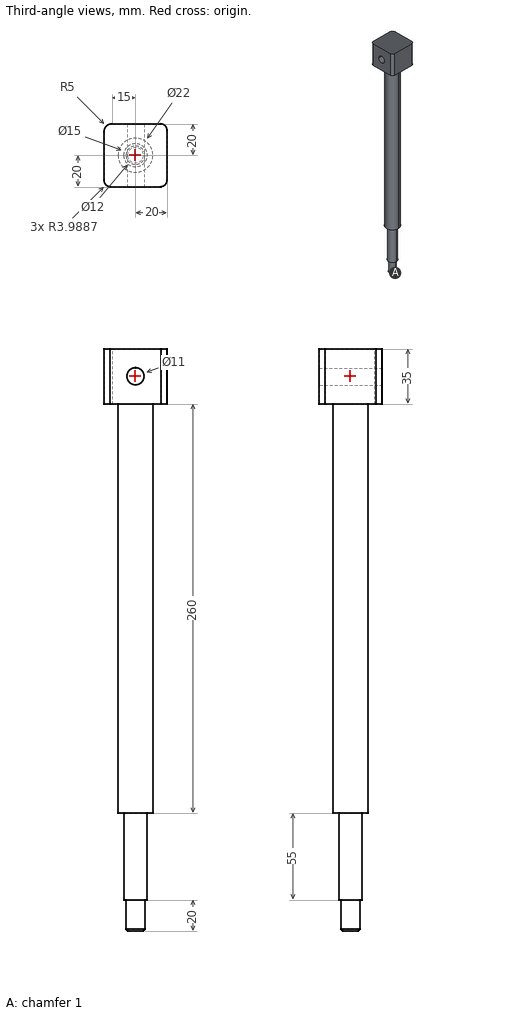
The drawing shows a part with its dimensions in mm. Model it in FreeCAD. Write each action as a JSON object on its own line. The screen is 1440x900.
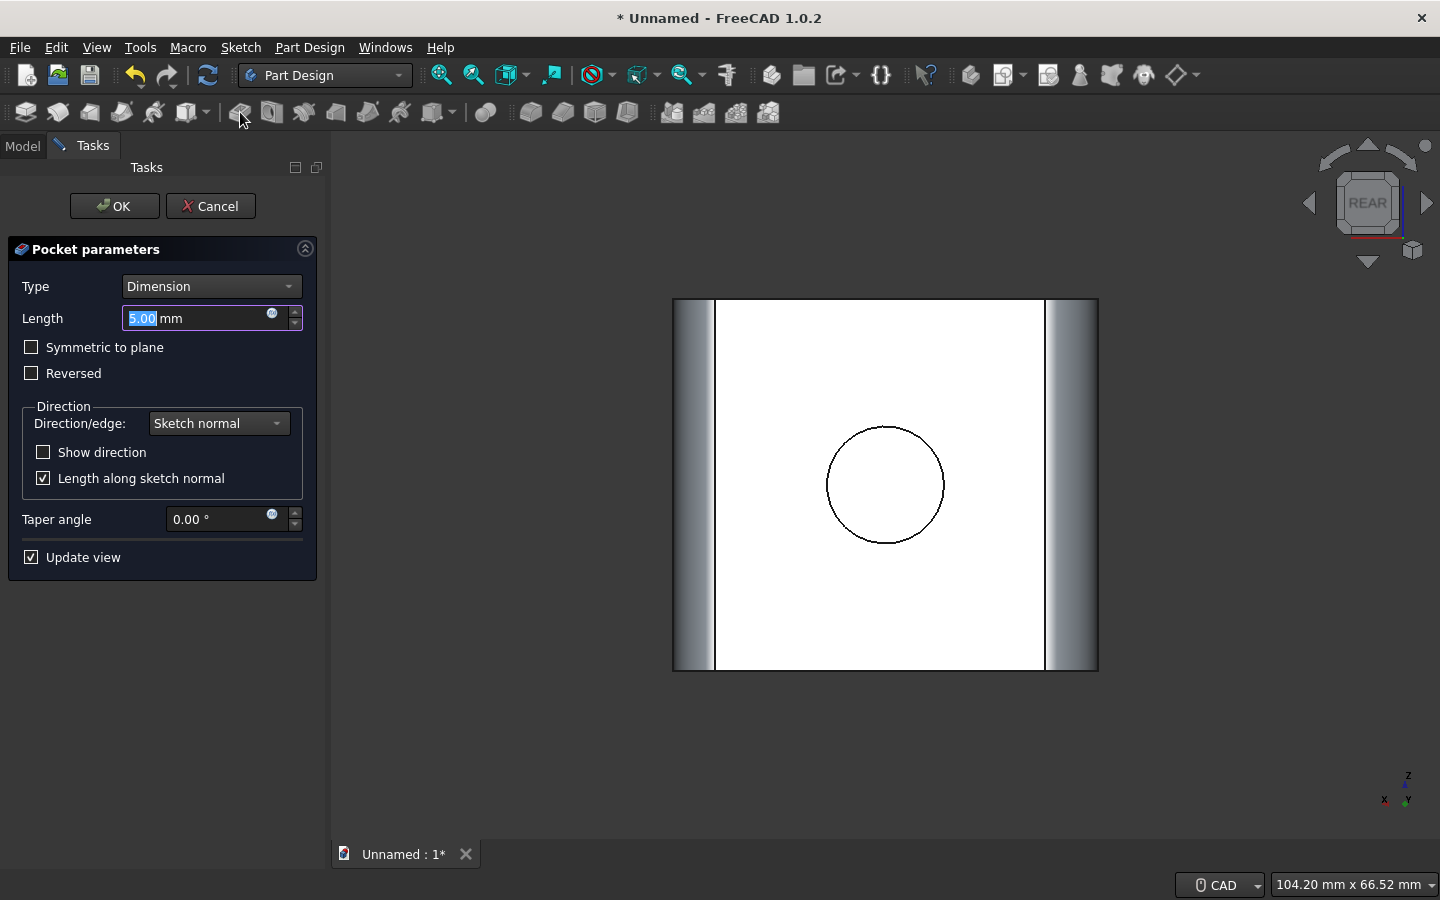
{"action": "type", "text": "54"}
{"action": "key", "text": "Tab"}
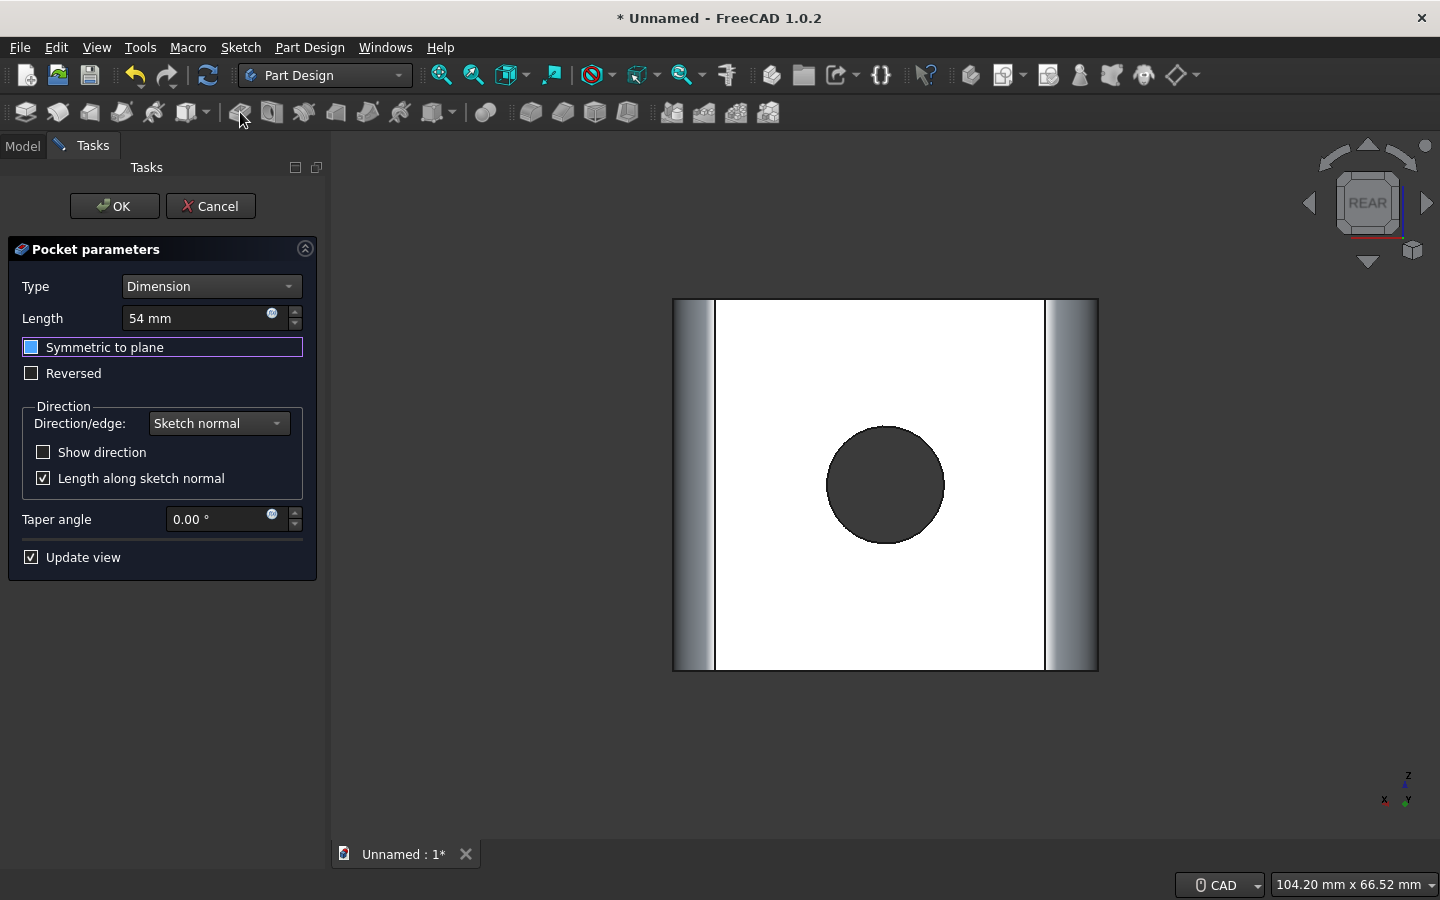
{"action": "left_click", "coordinate": [115, 206]}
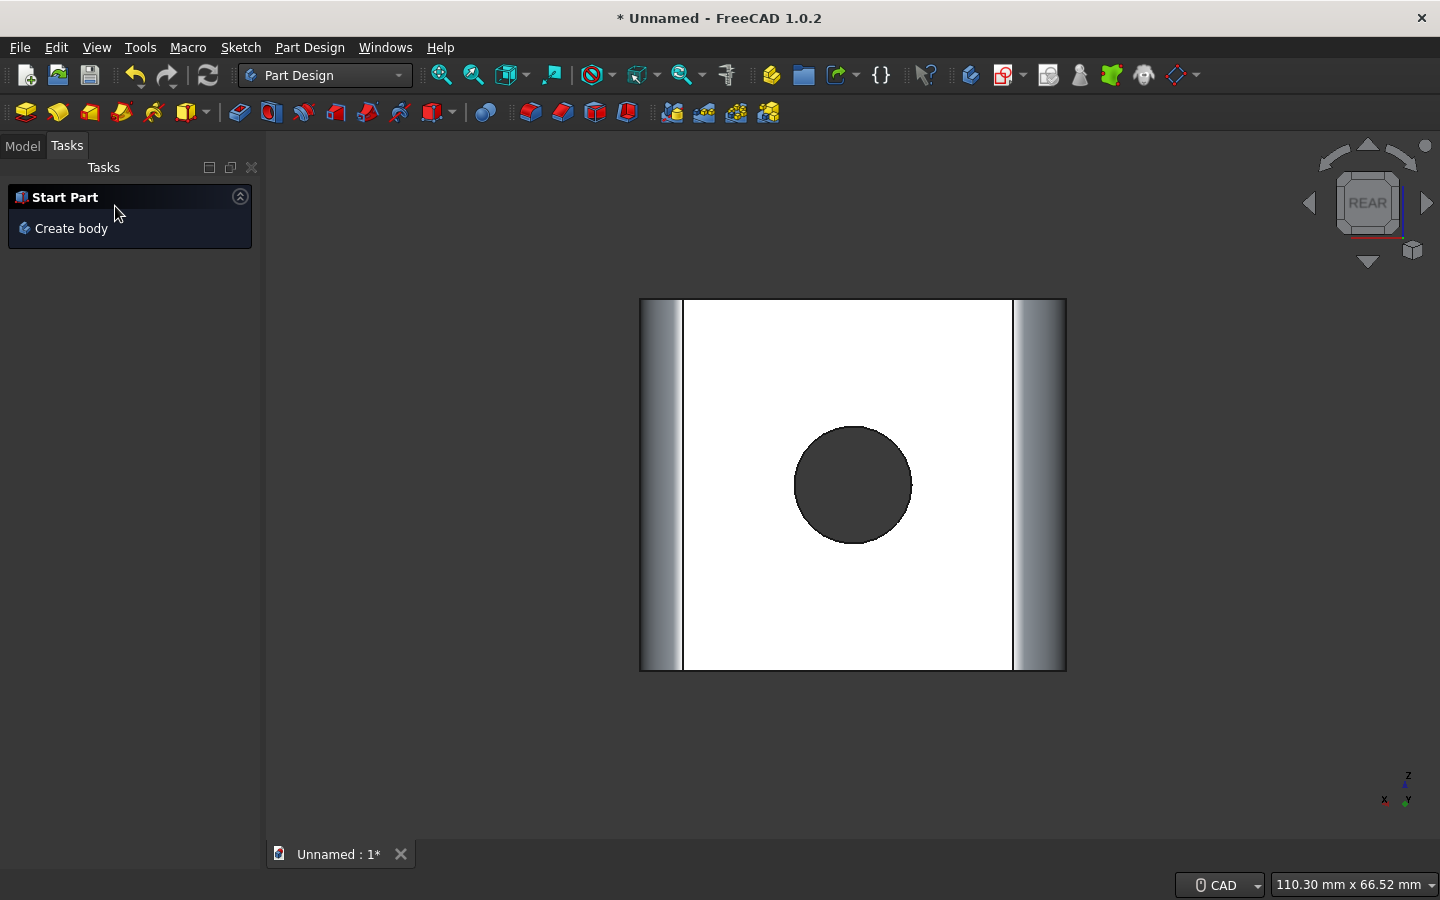
{"action": "key", "text": "5"}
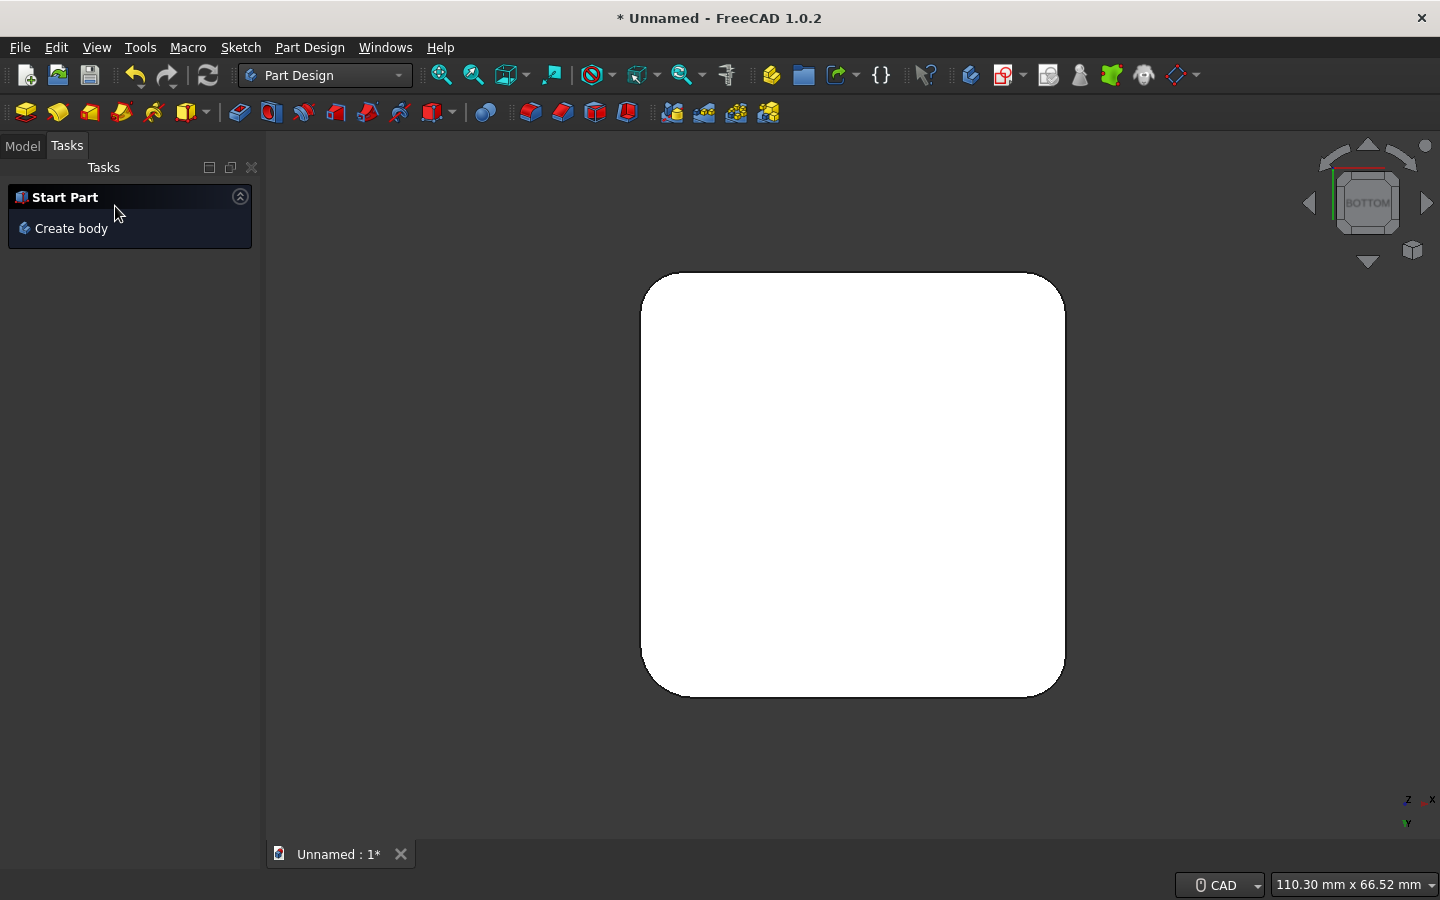
{"action": "left_click", "coordinate": [853, 484]}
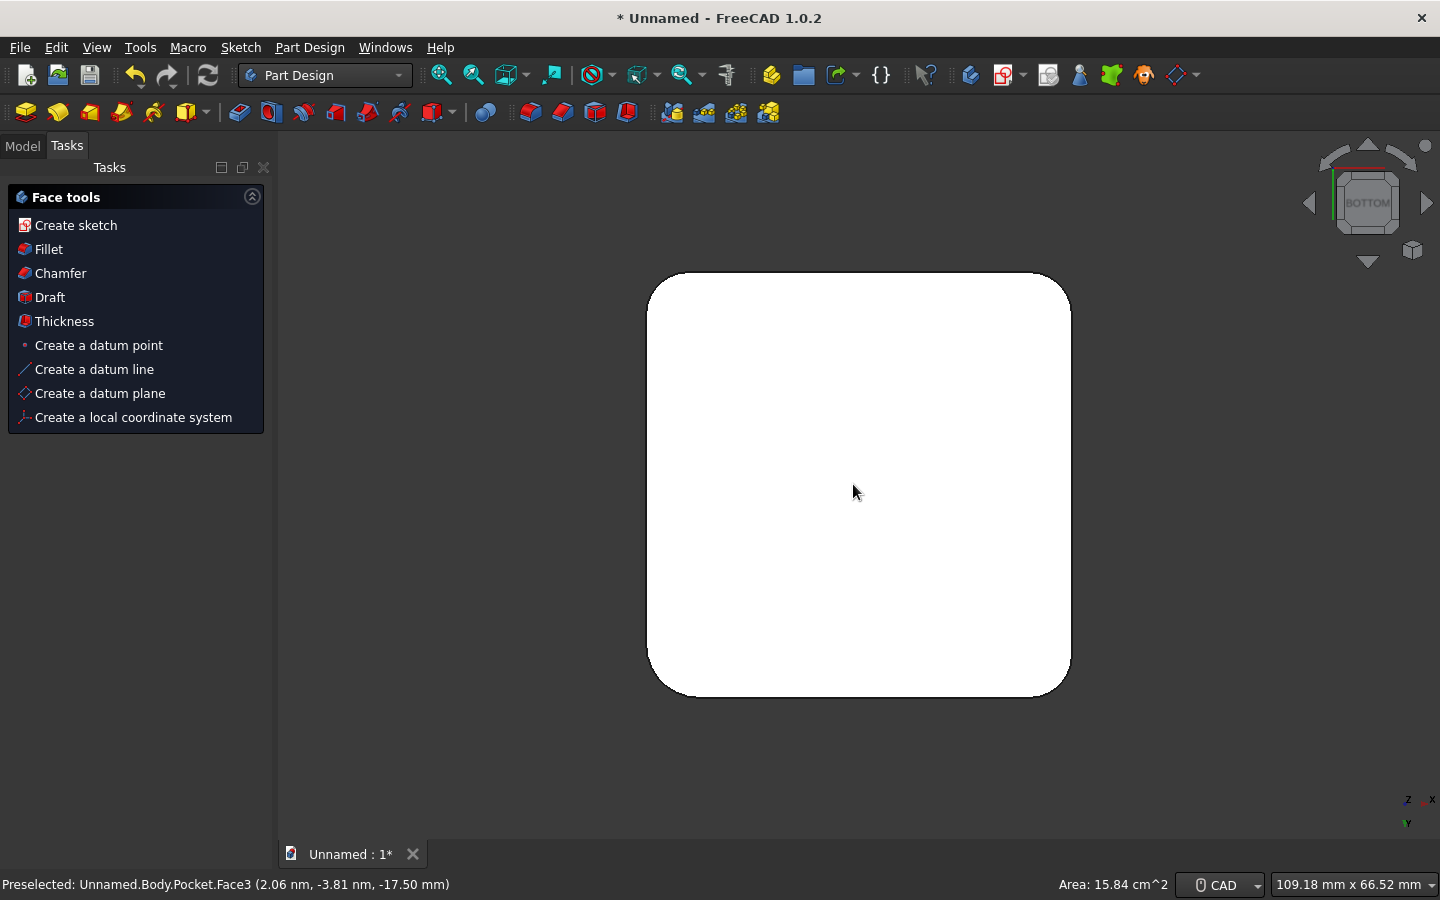
{"action": "left_click", "coordinate": [1004, 76]}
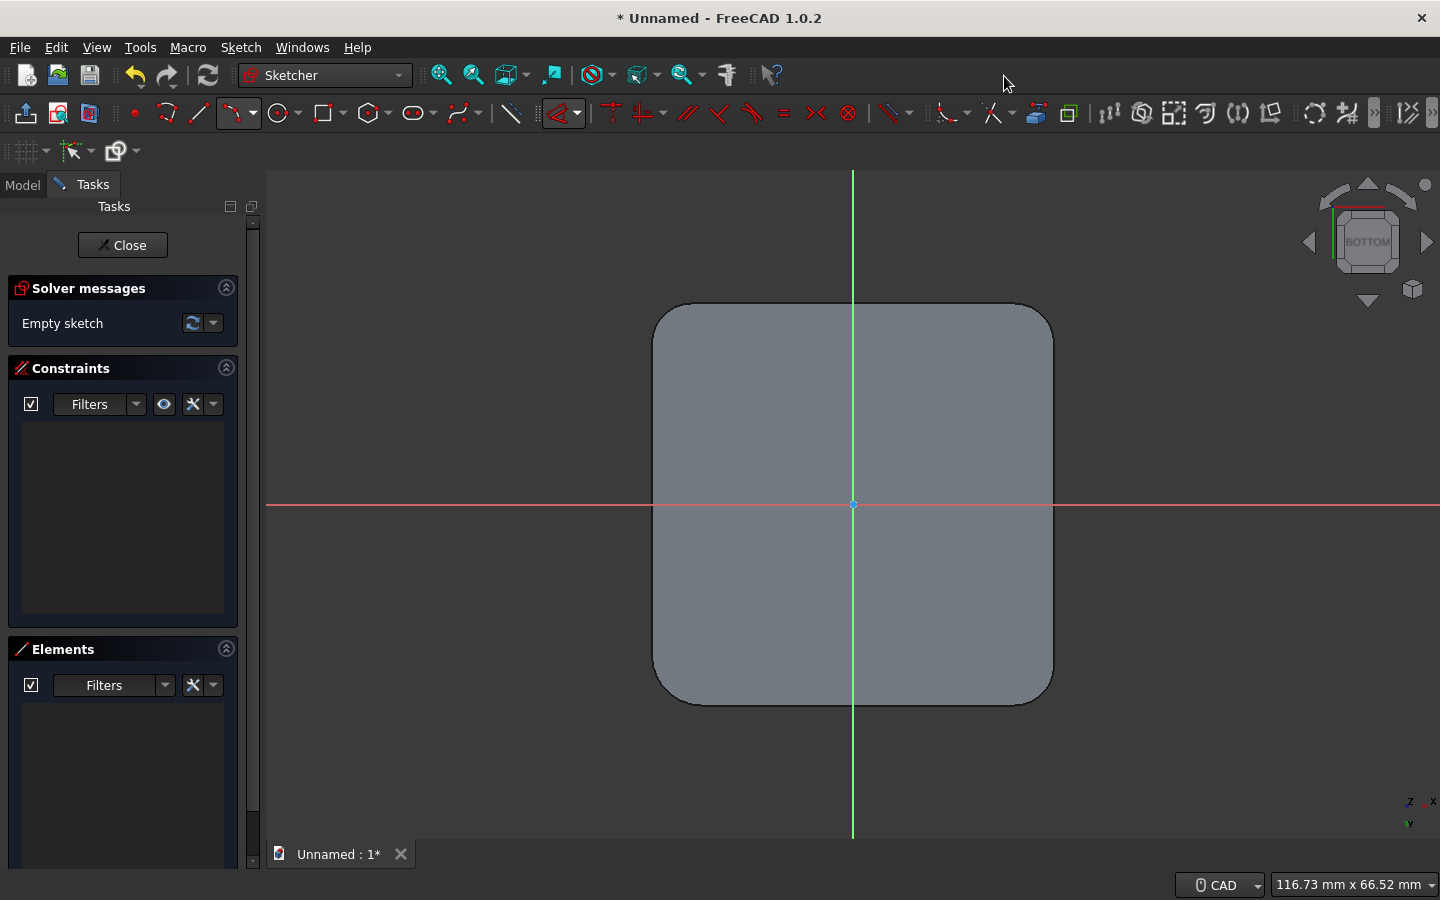
{"action": "scroll", "coordinate": [936, 505], "scroll_direction": "up", "scroll_amount": 3}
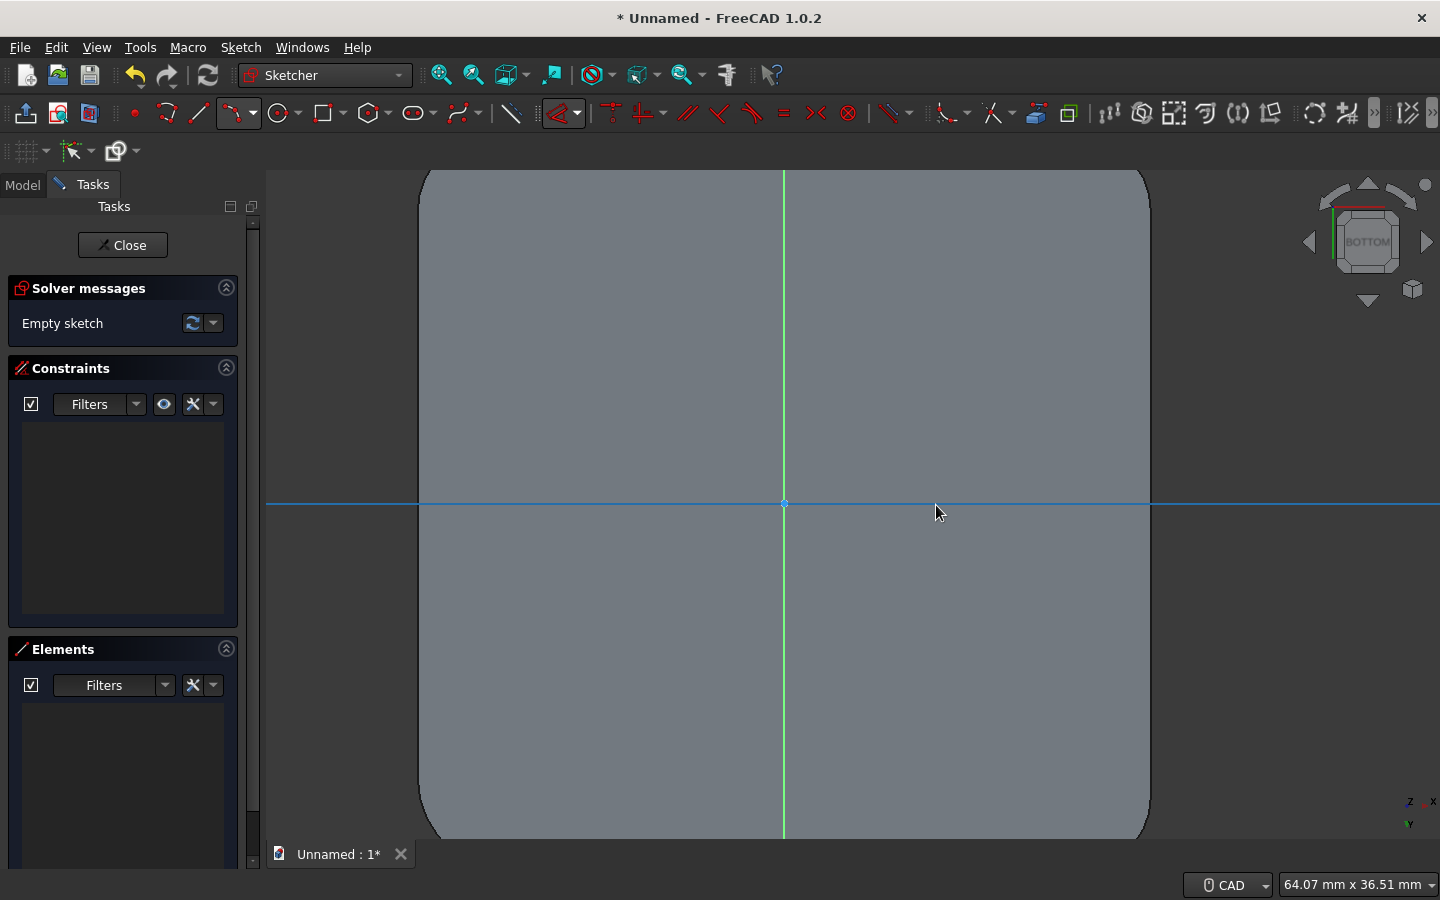
{"action": "left_click", "coordinate": [278, 114]}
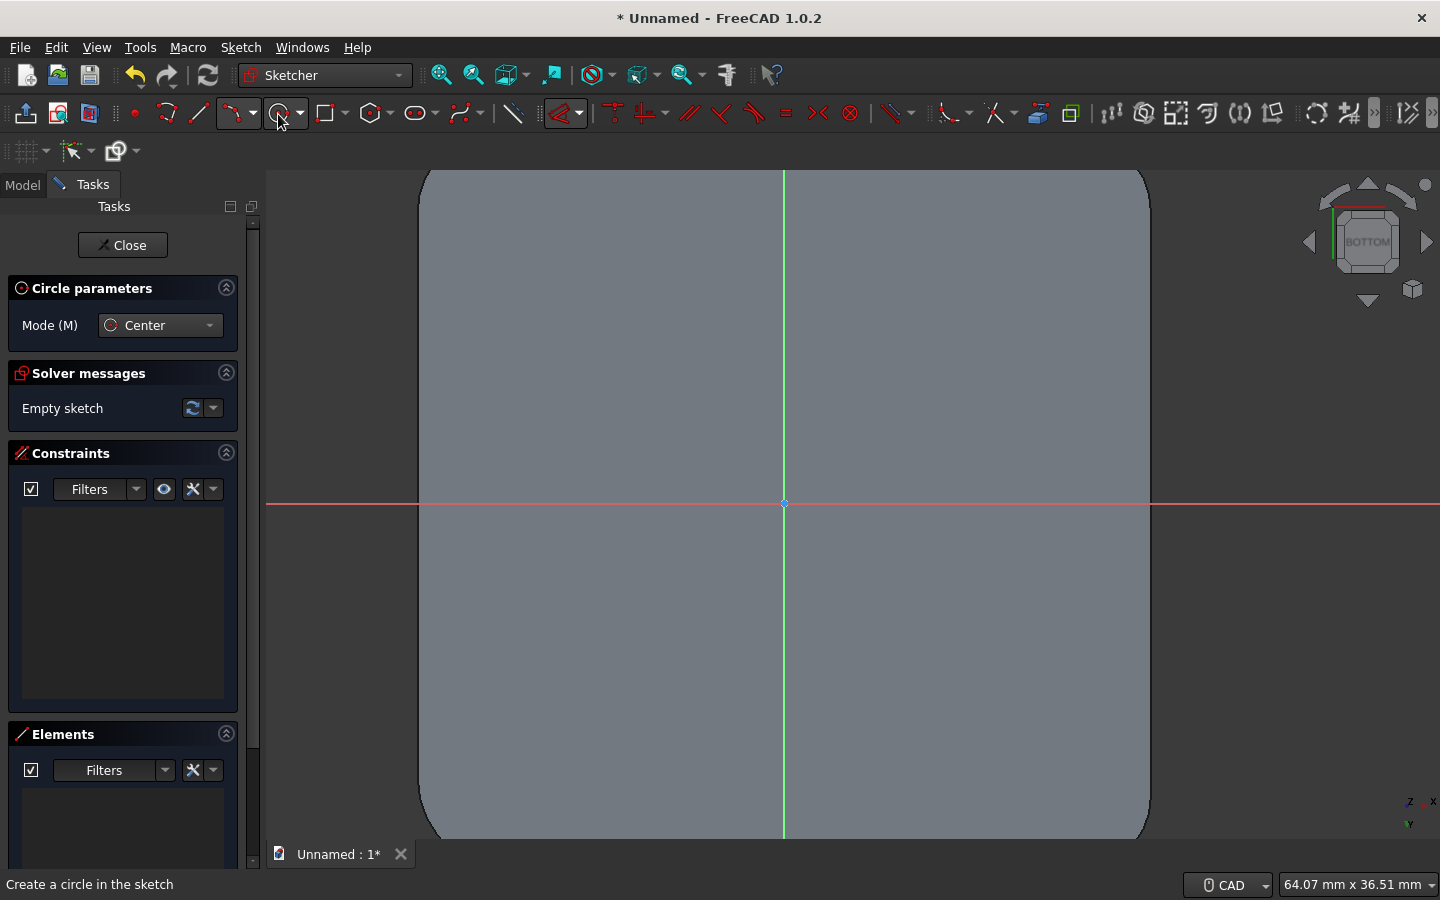
{"action": "left_click", "coordinate": [784, 504]}
{"action": "left_click", "coordinate": [927, 361]}
{"action": "key", "text": "Escape"}